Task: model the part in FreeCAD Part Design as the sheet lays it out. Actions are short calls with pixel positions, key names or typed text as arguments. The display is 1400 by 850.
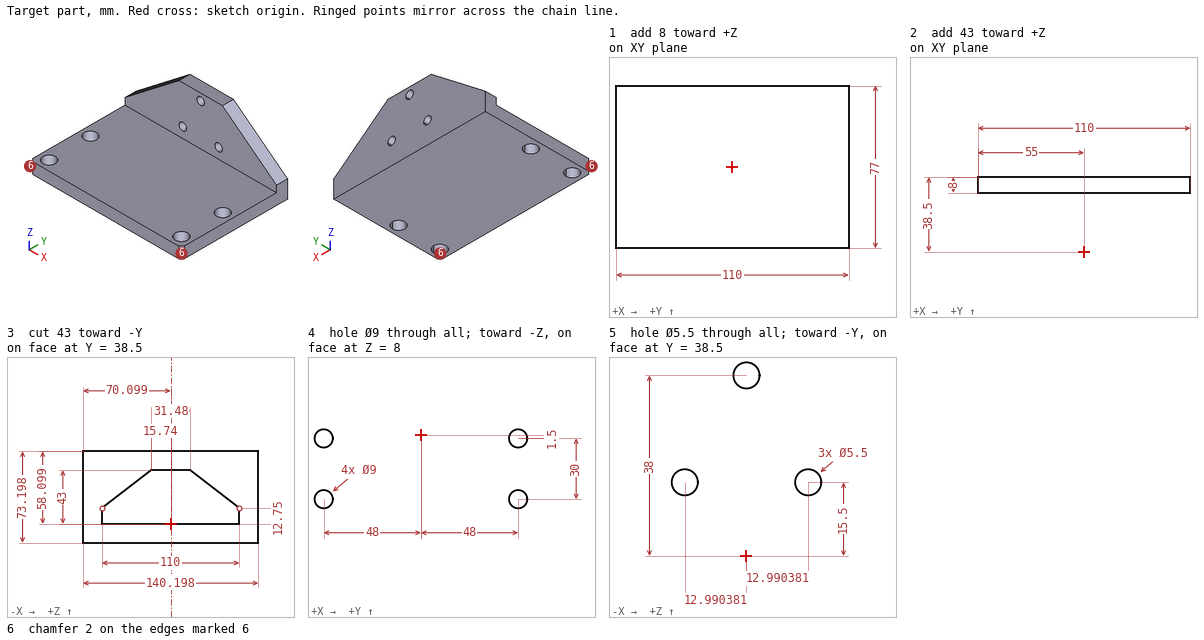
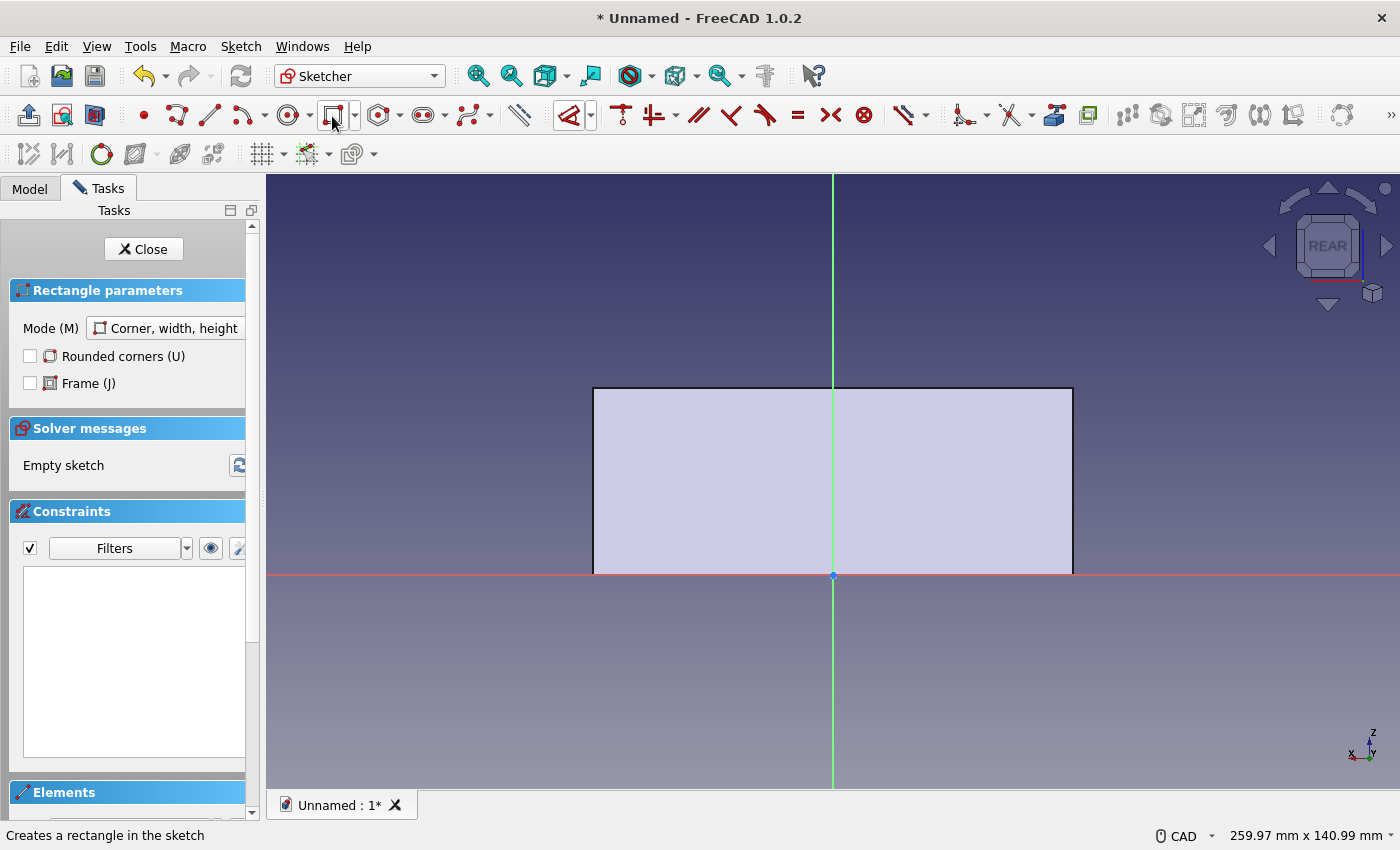
click(527, 322)
click(1139, 641)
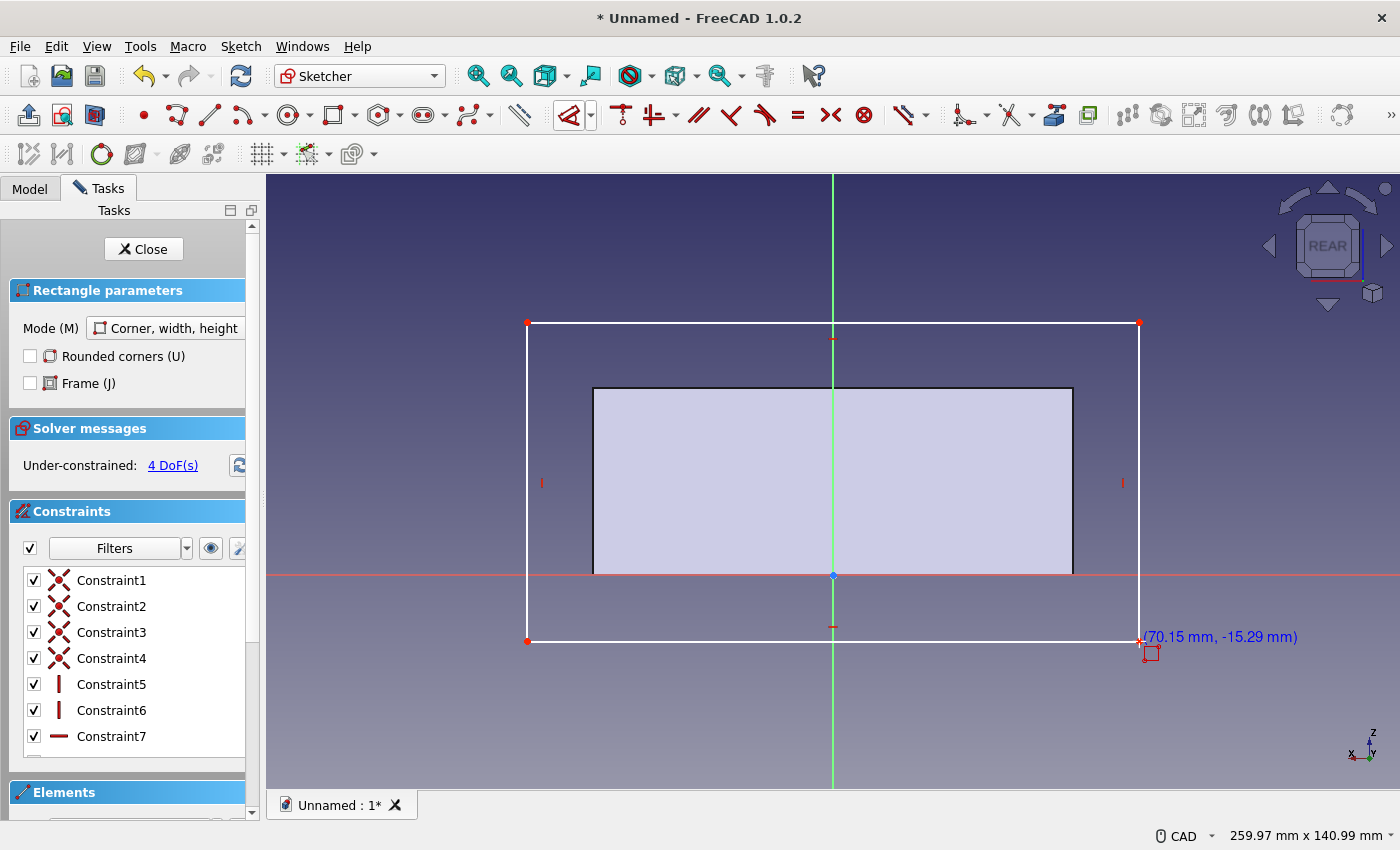
key(g)
key(m)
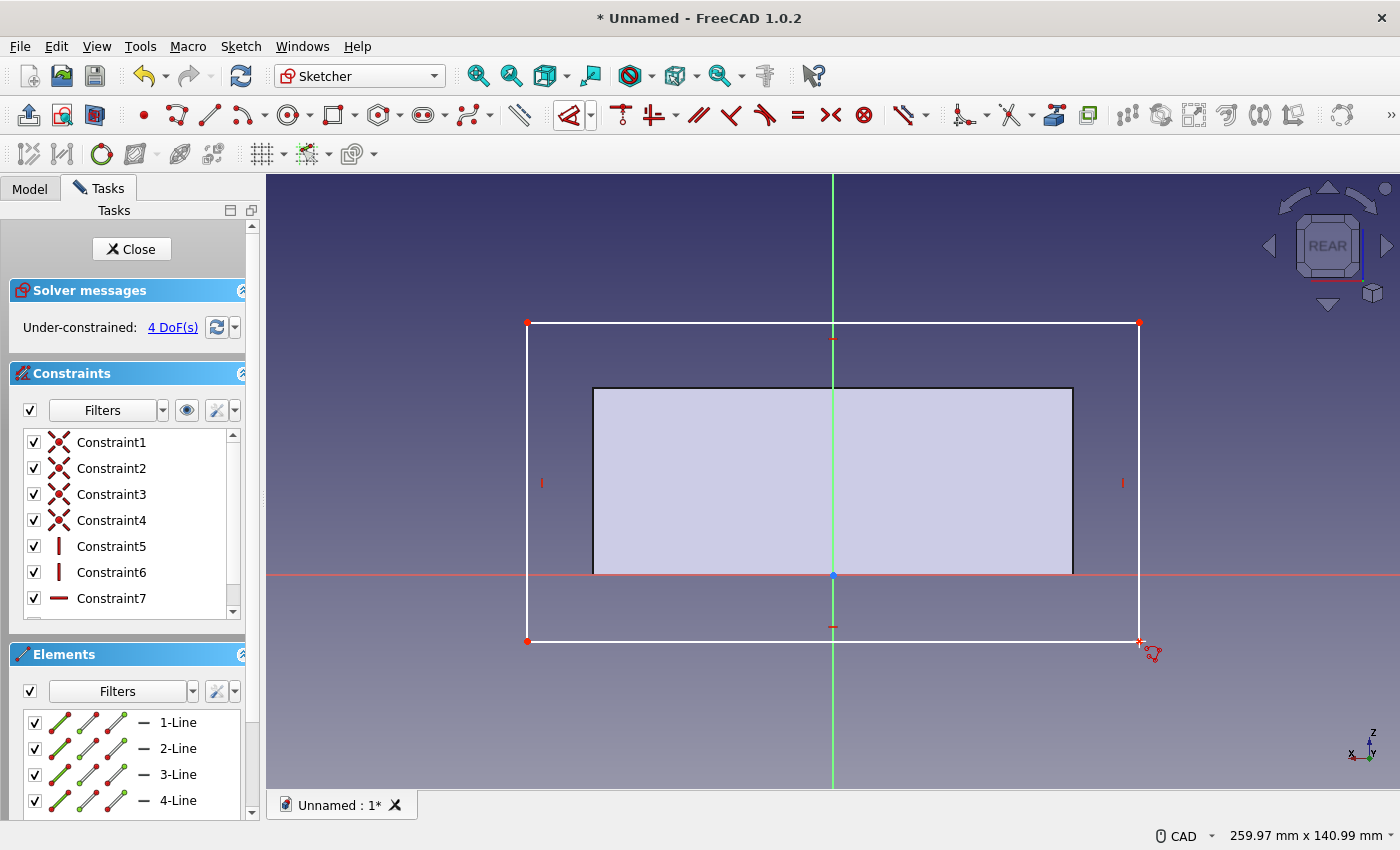
click(764, 388)
click(902, 388)
click(1073, 520)
click(1073, 575)
click(593, 566)
click(593, 520)
click(764, 389)
key(Escape)
key(Escape)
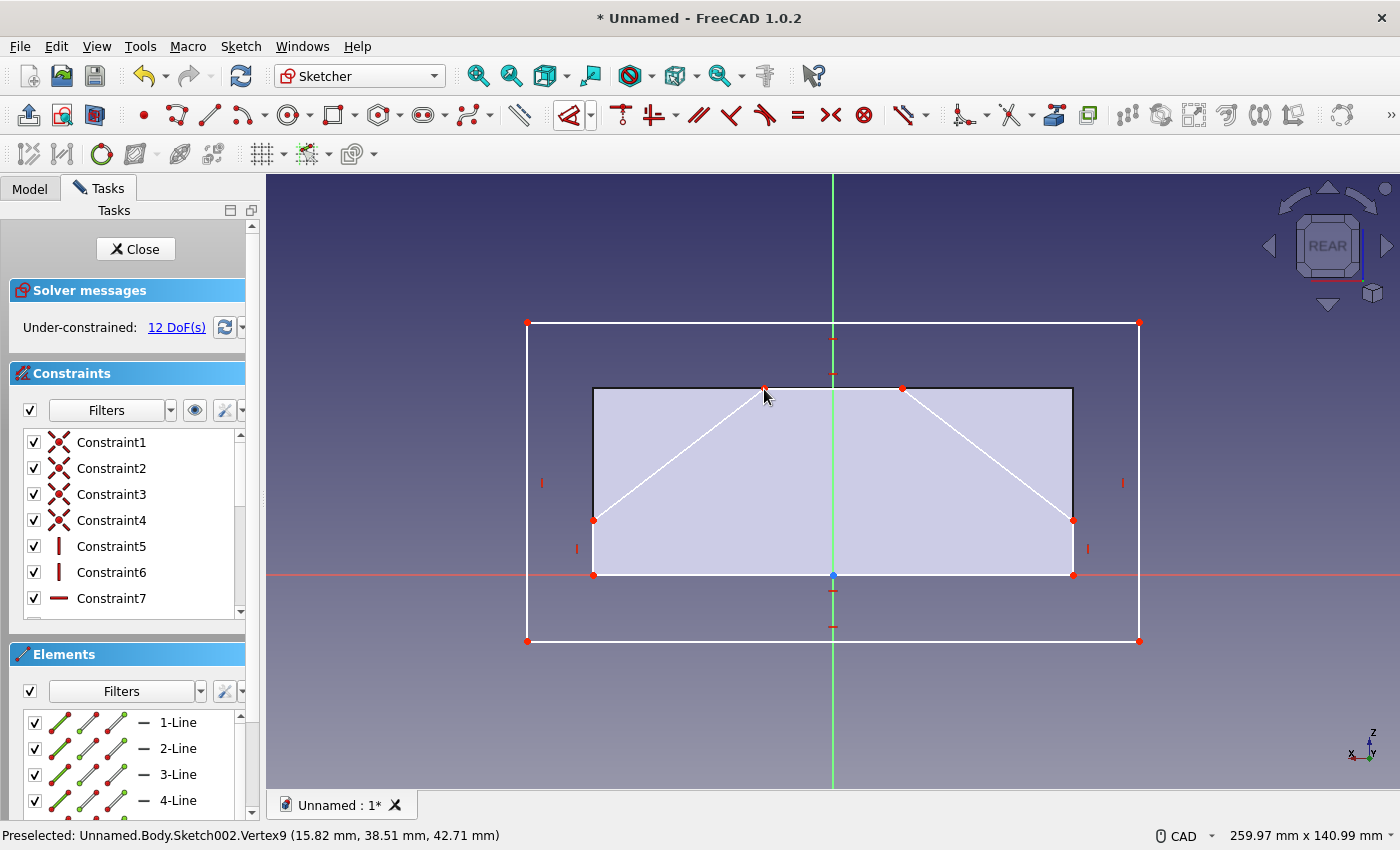
click(1073, 521)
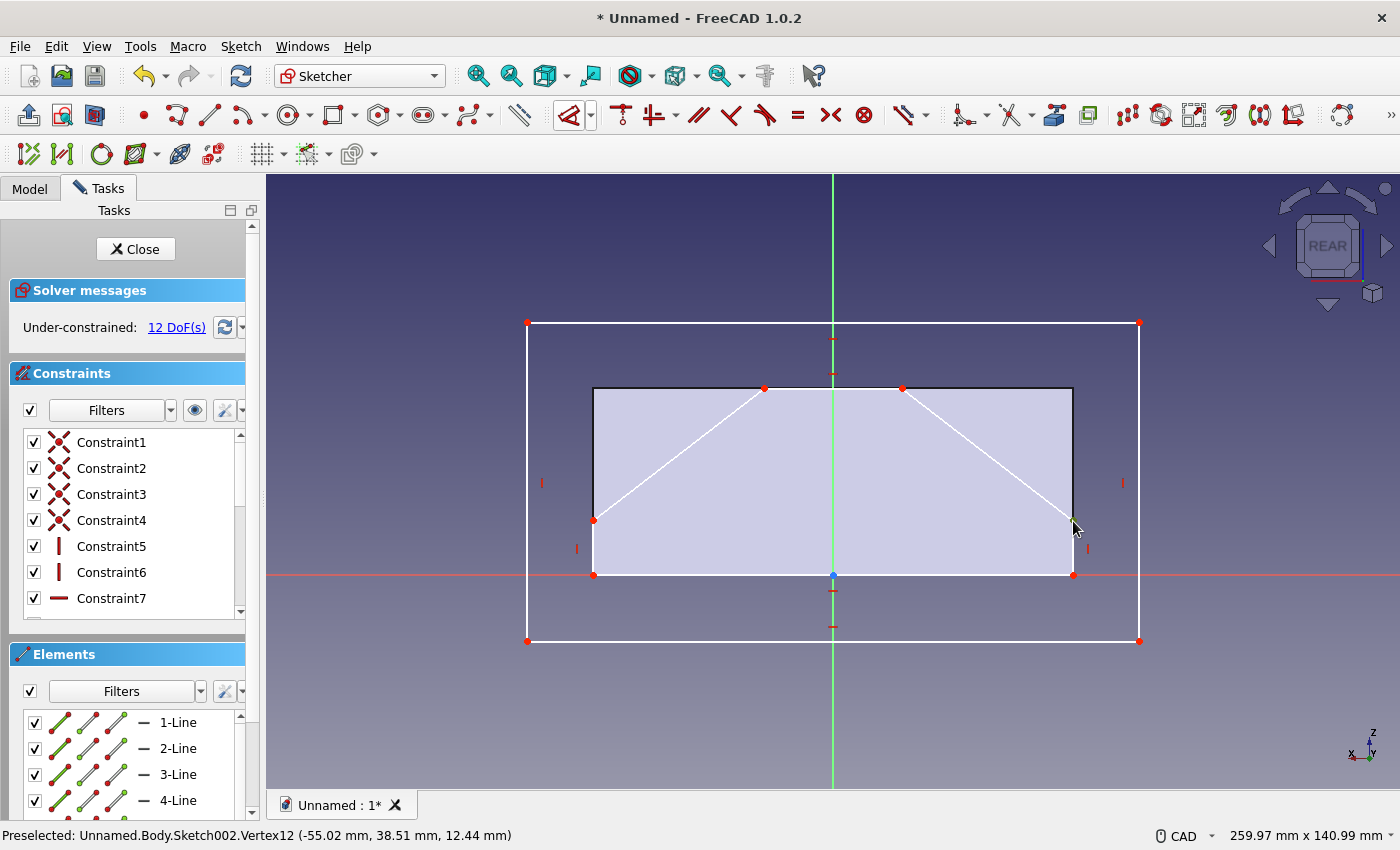
click(593, 521)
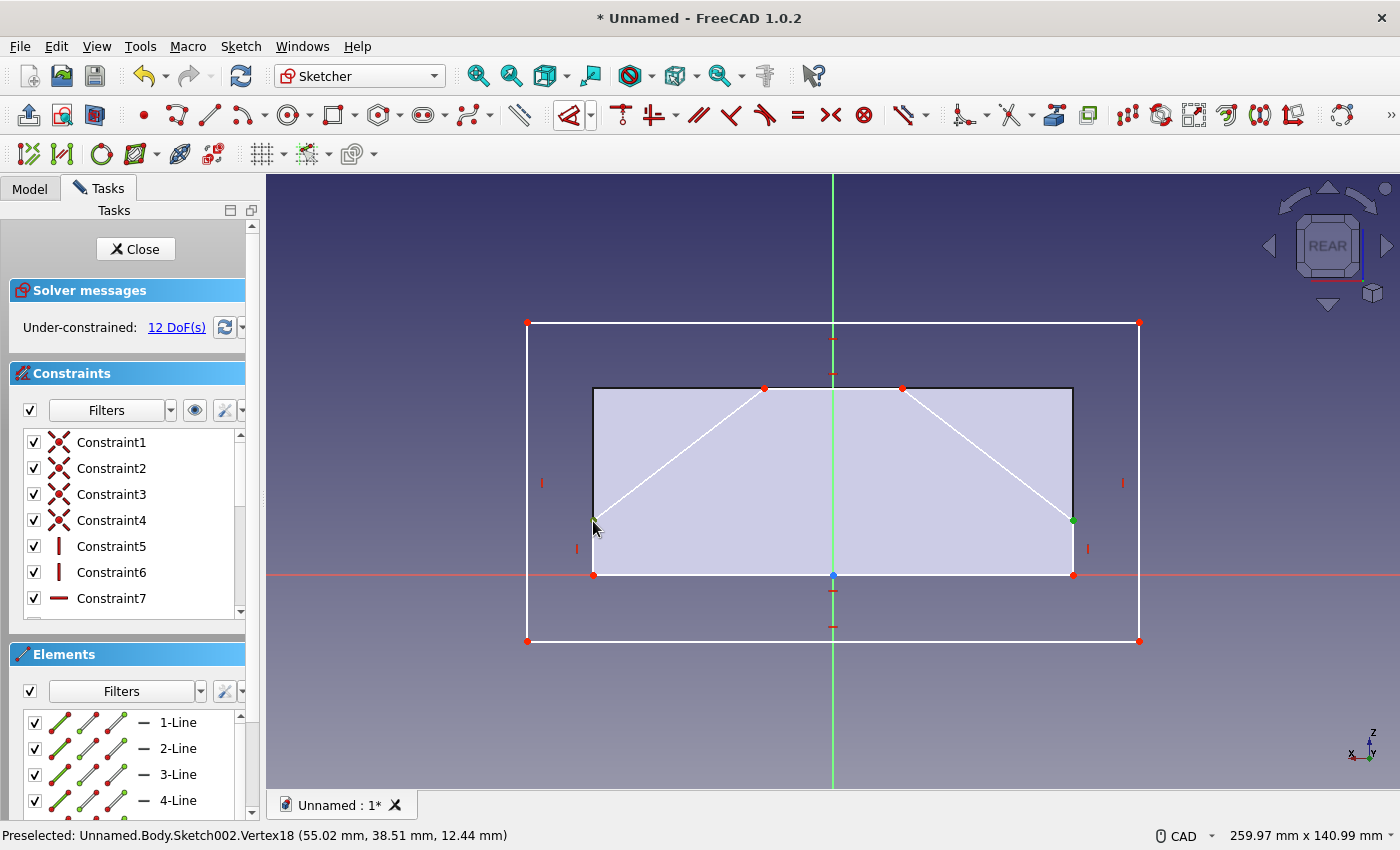
click(833, 721)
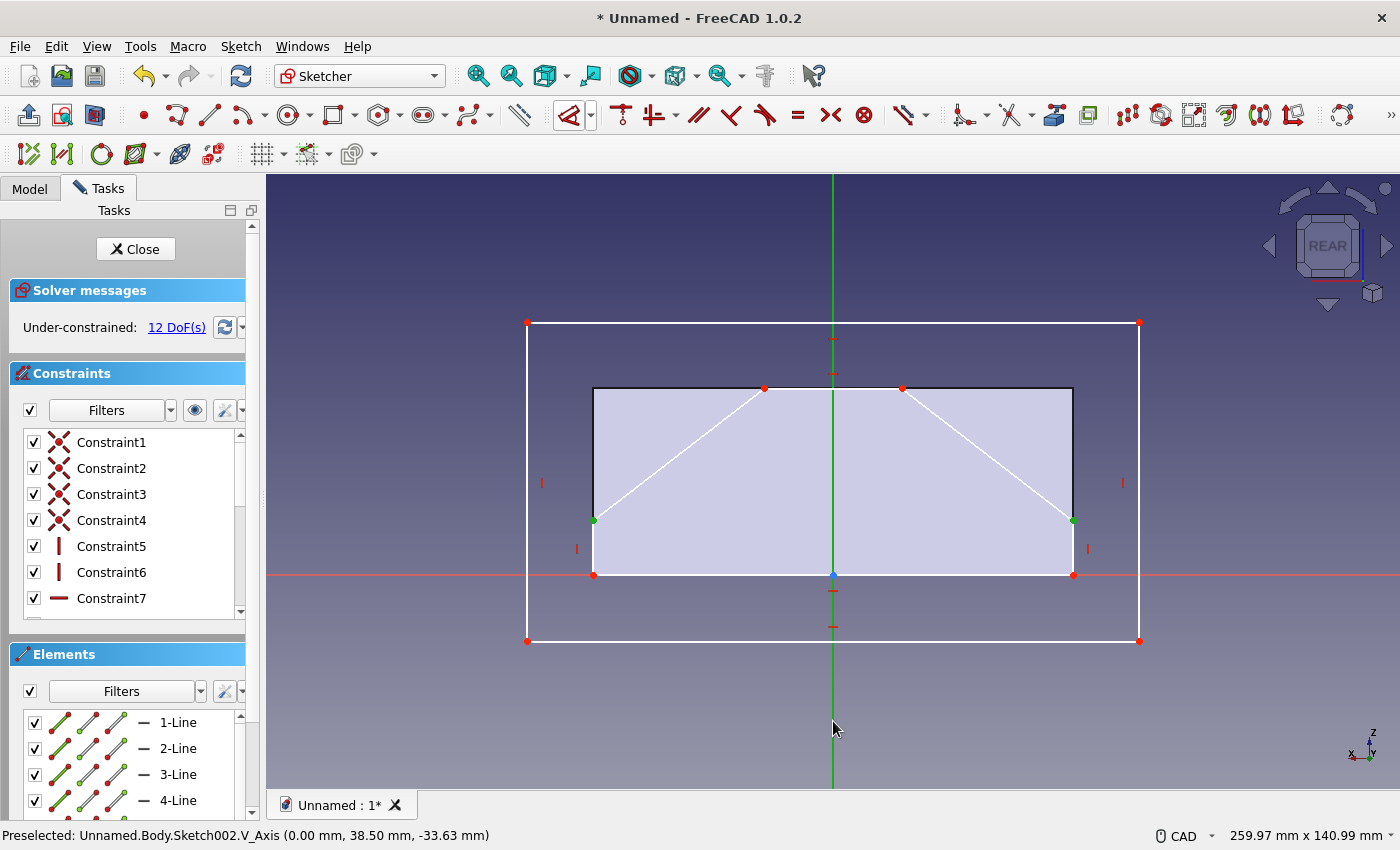
click(831, 116)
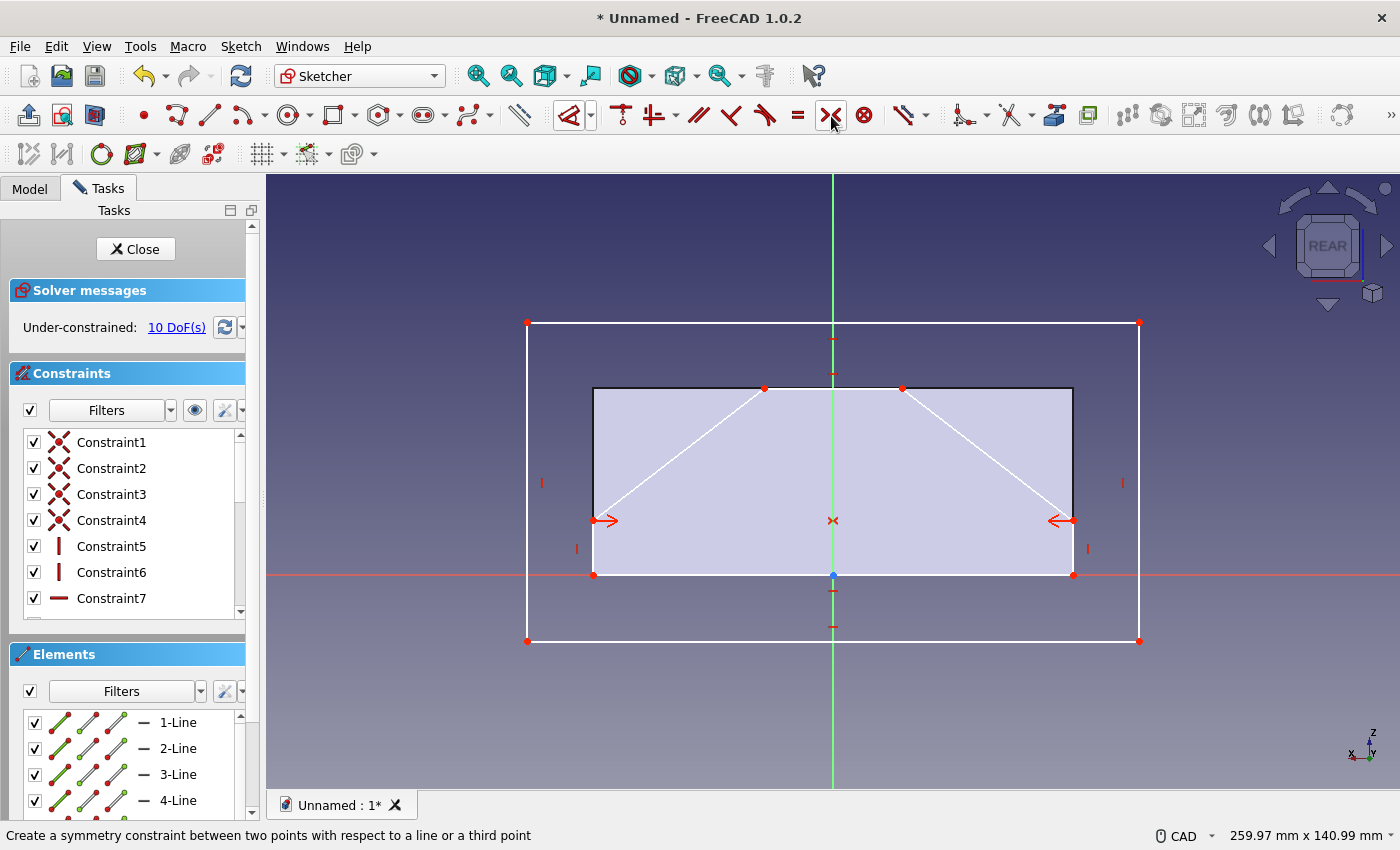
click(1073, 575)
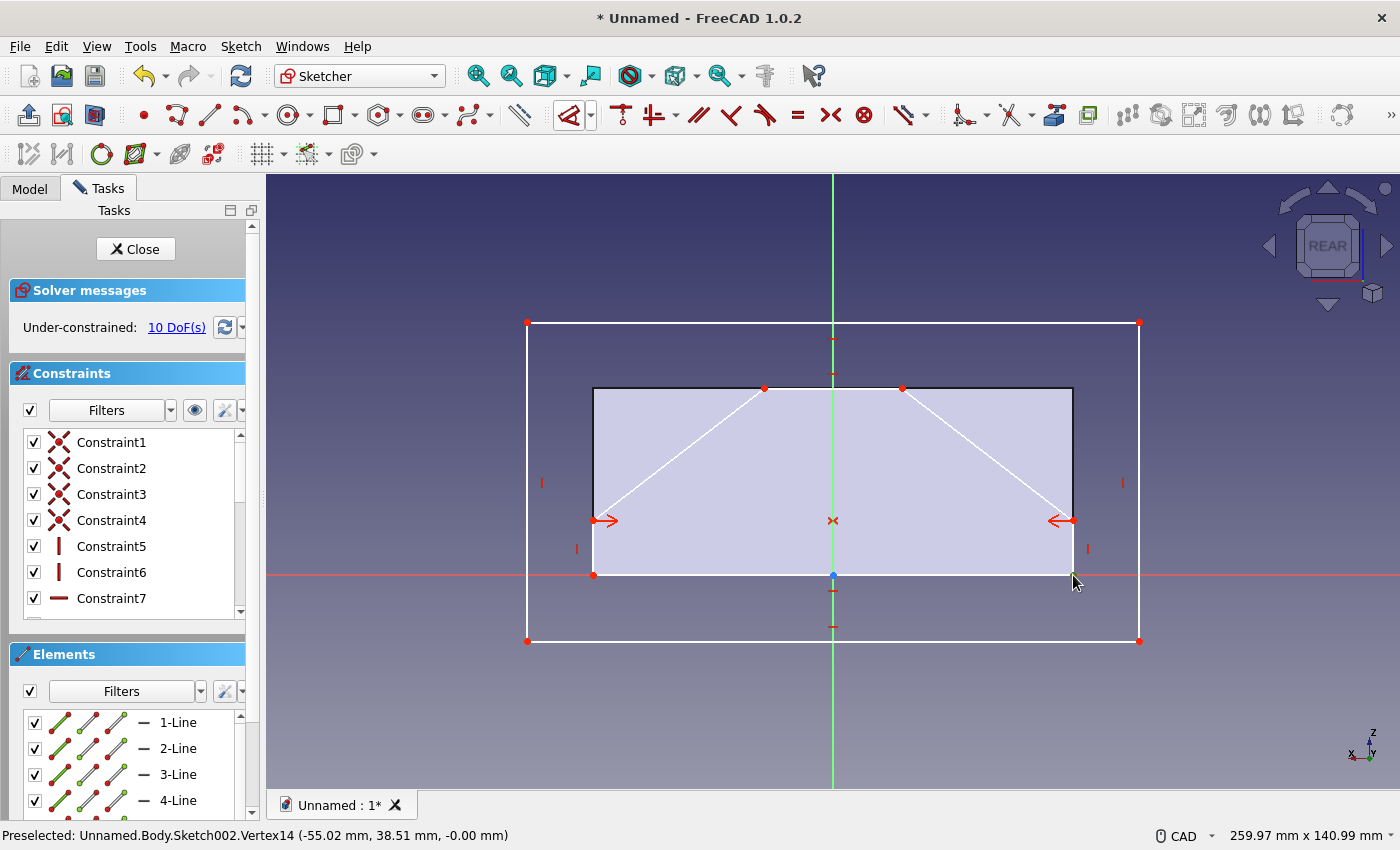
click(361, 575)